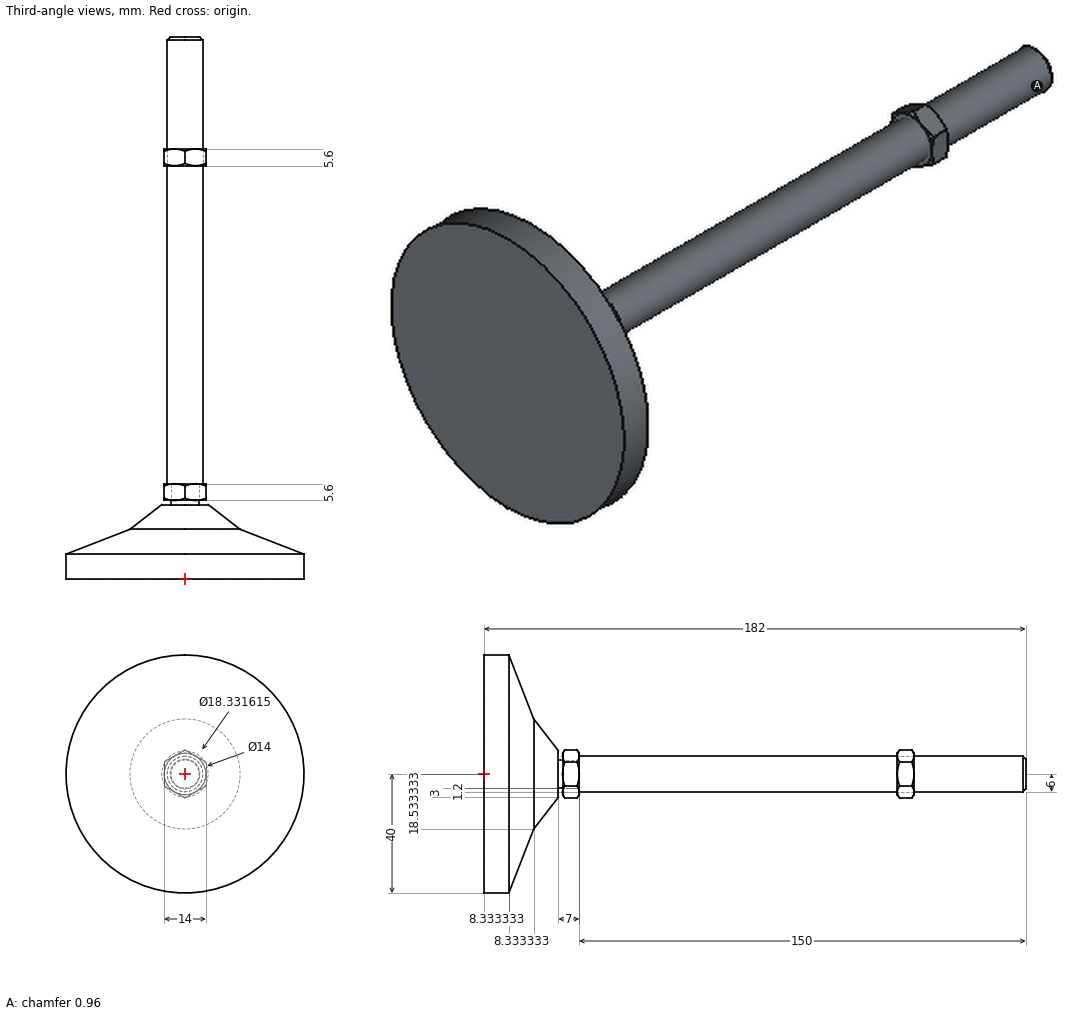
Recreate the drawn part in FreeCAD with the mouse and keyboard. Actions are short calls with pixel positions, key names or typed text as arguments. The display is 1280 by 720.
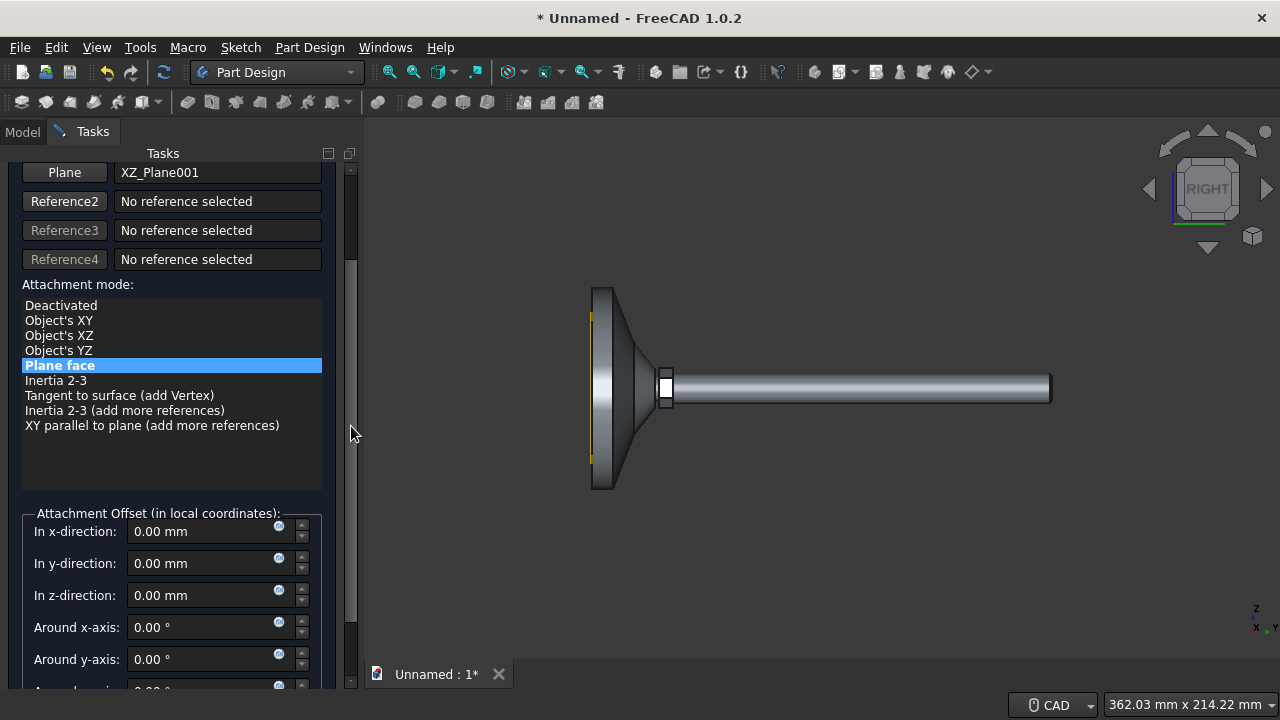
triple_click(210, 595)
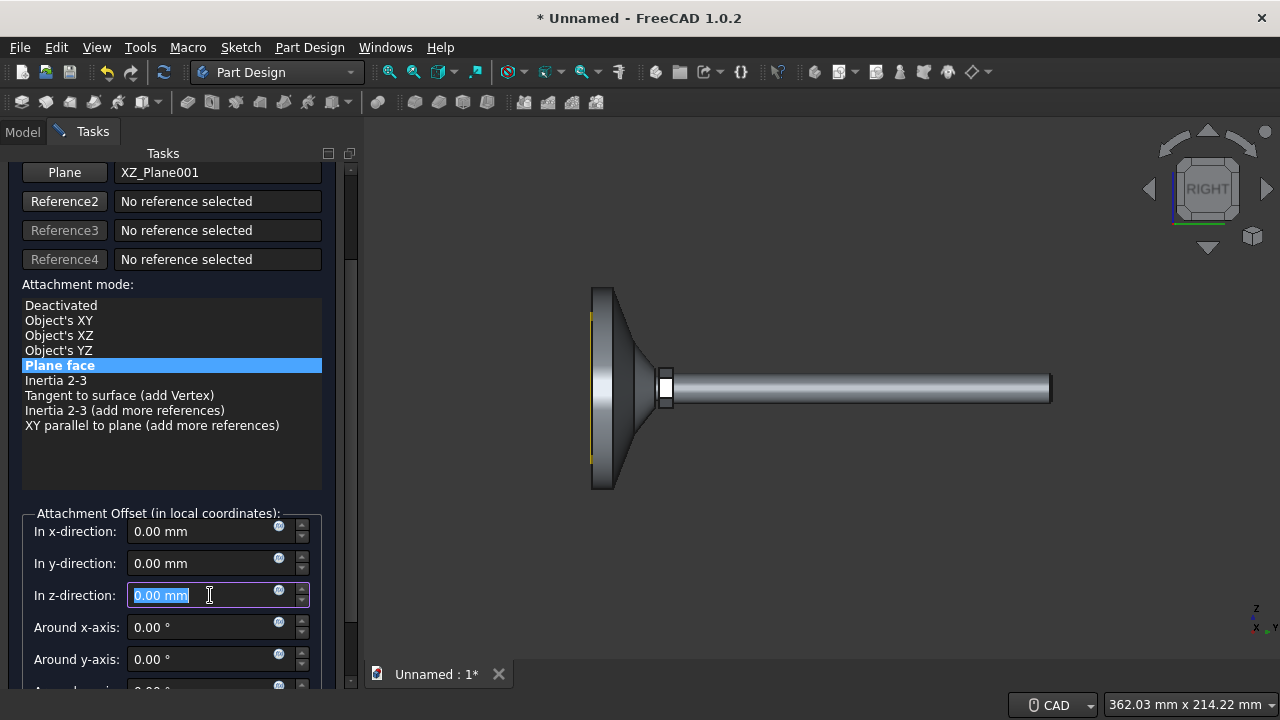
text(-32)
key(Tab)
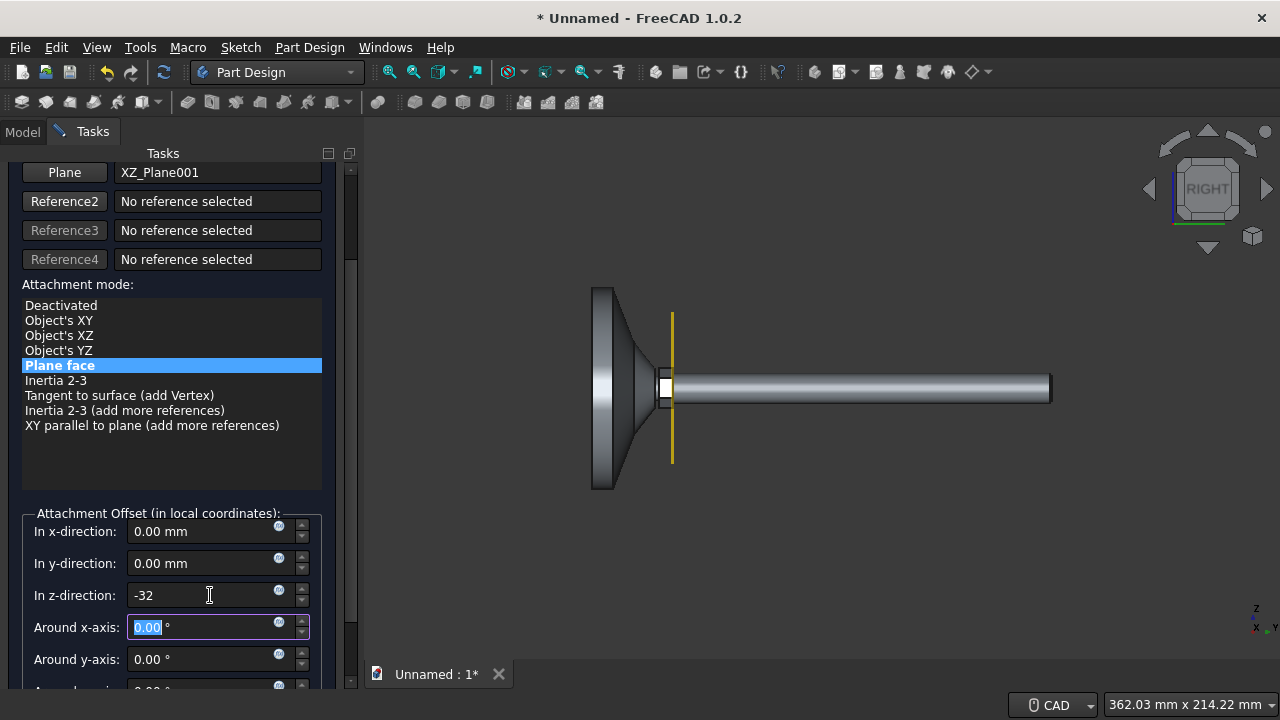
scroll(351, 426, up, 3)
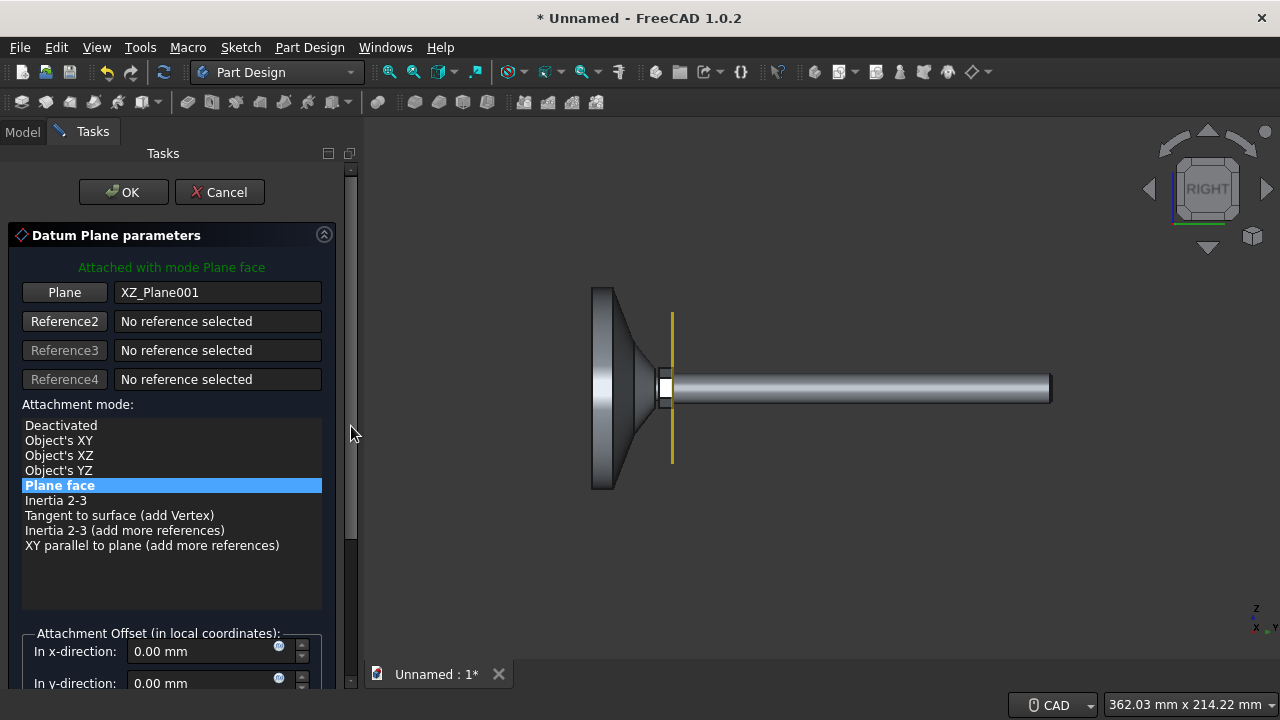
click(124, 192)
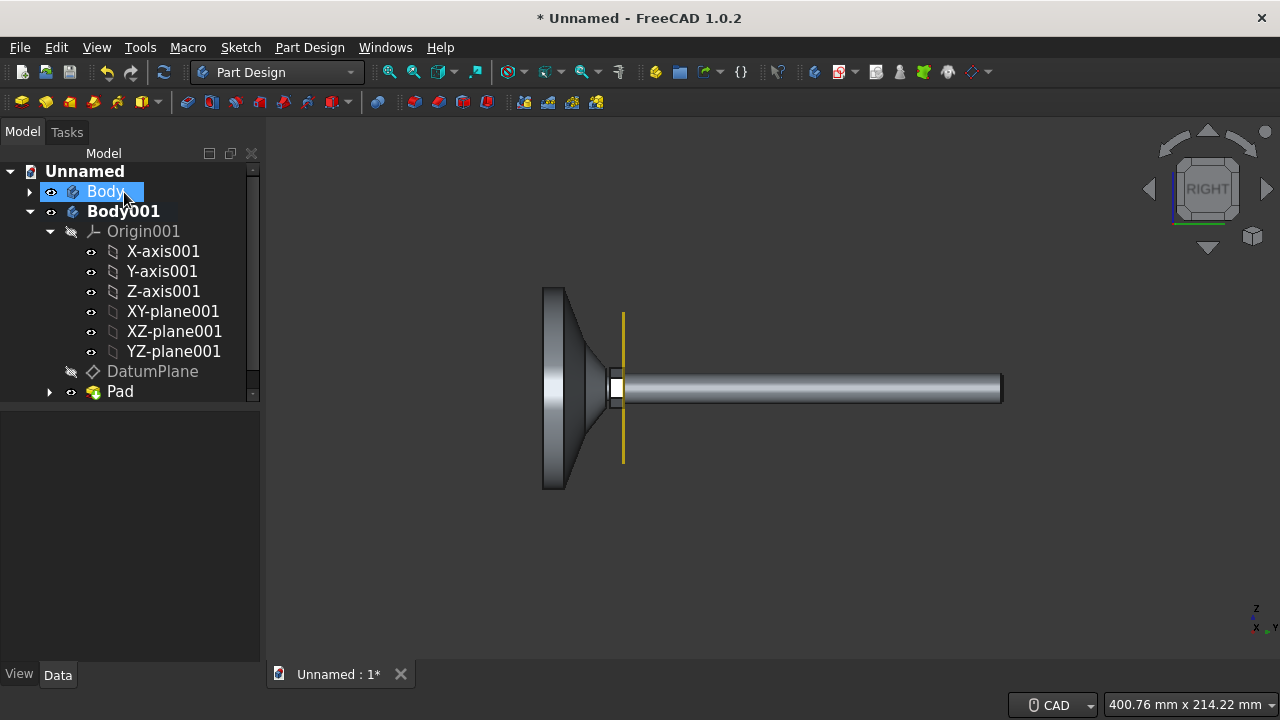
scroll(100, 287, down, 3)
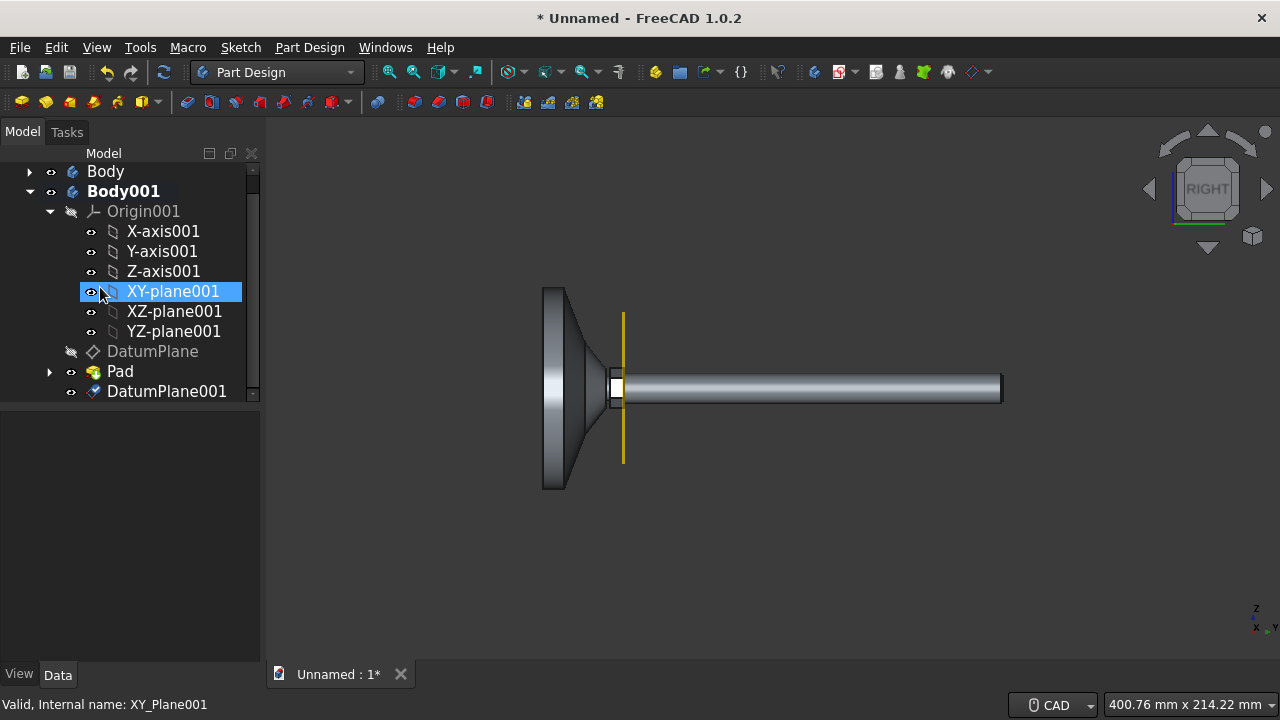
click(116, 392)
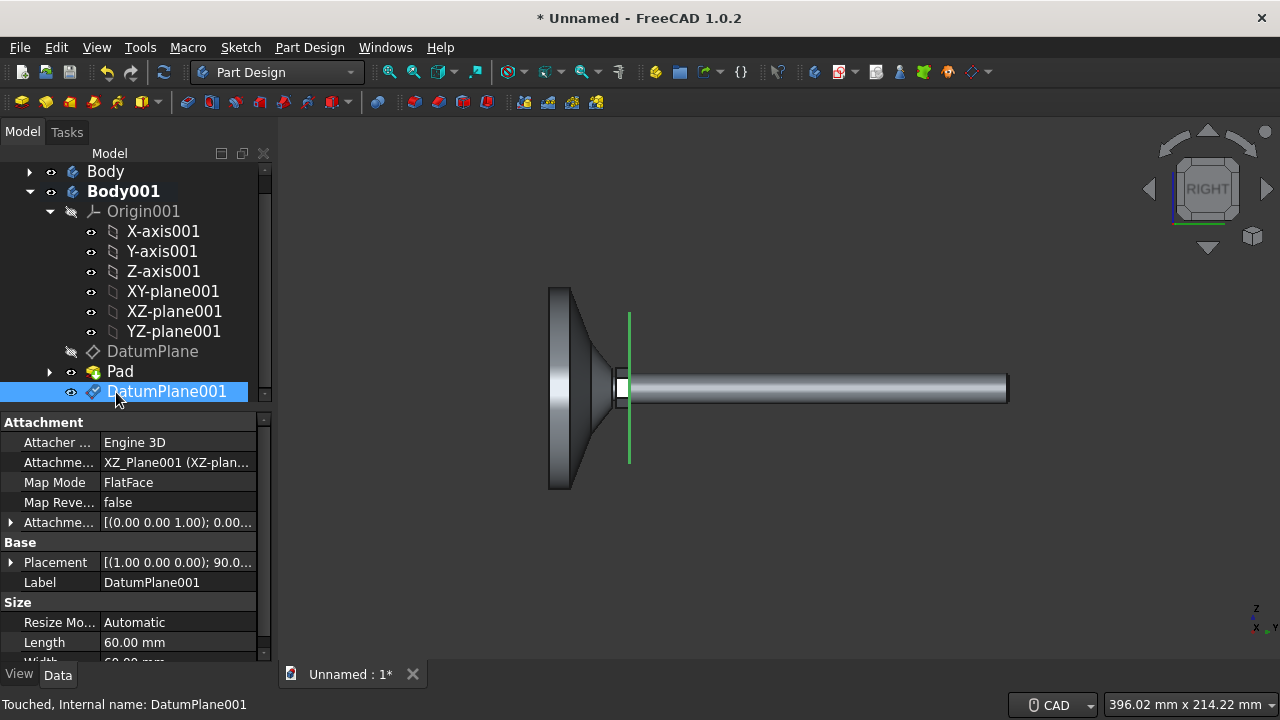
click(840, 72)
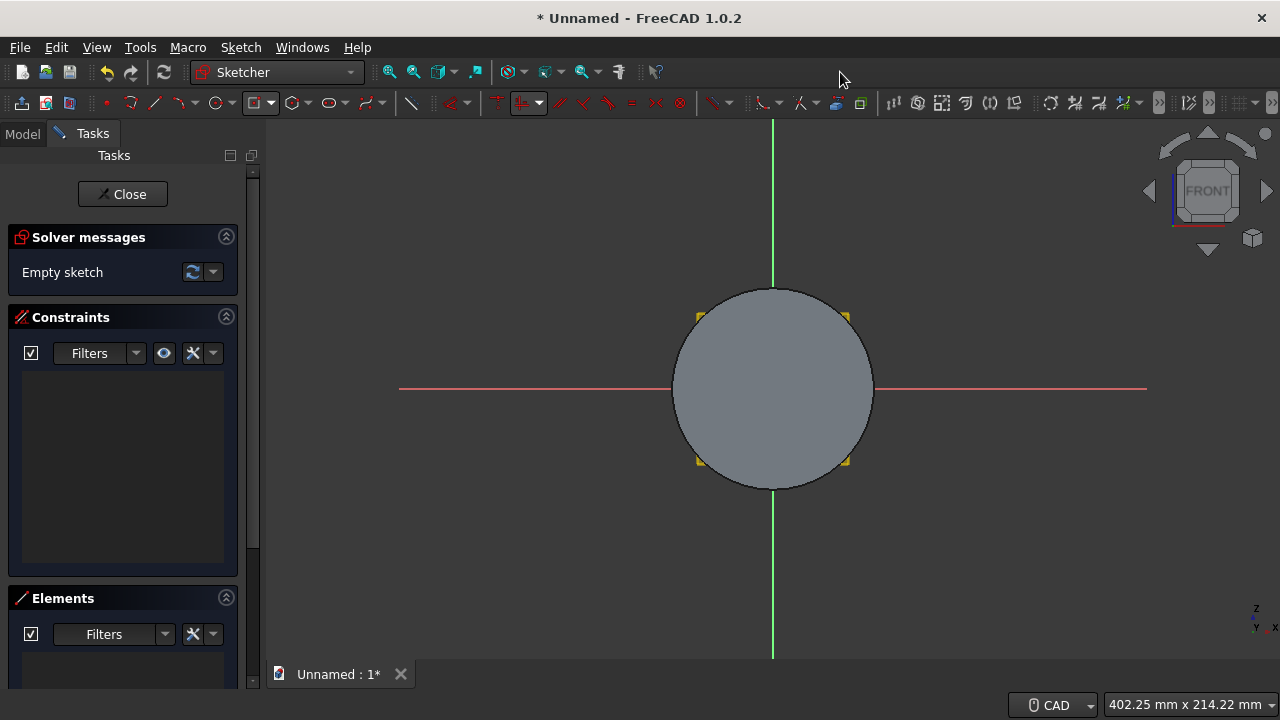
click(70, 104)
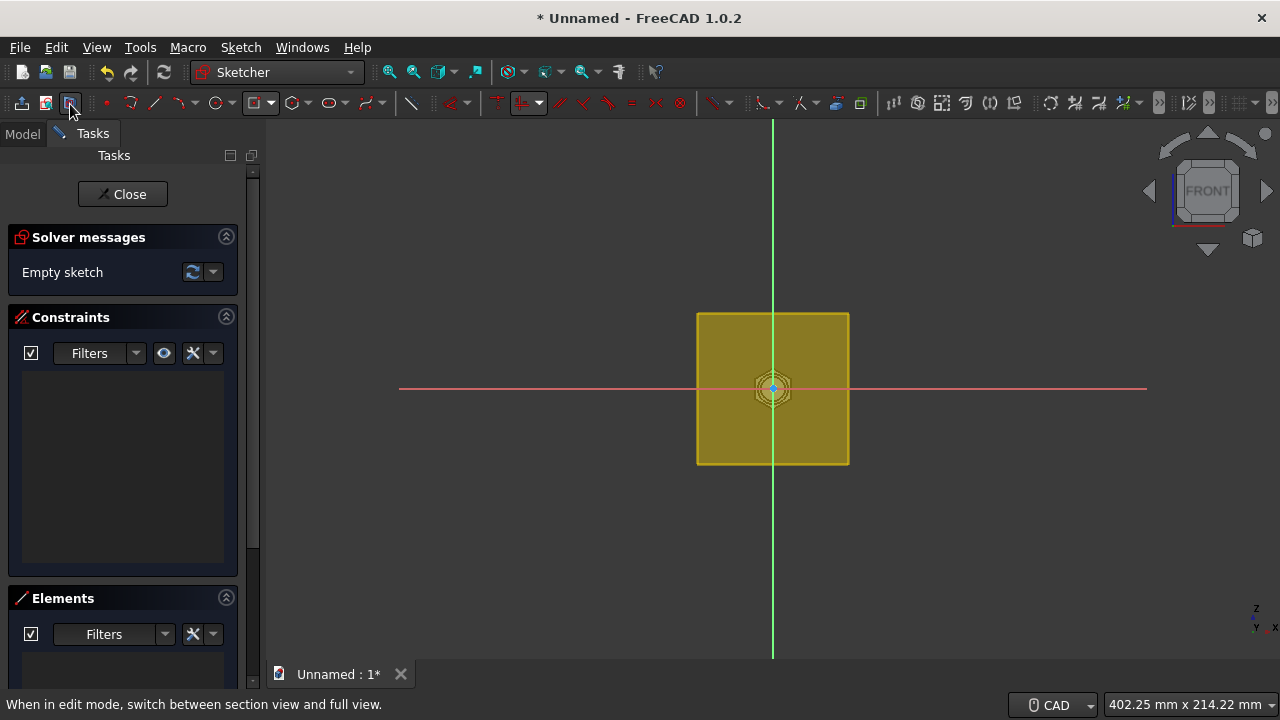
scroll(784, 389, up, 10)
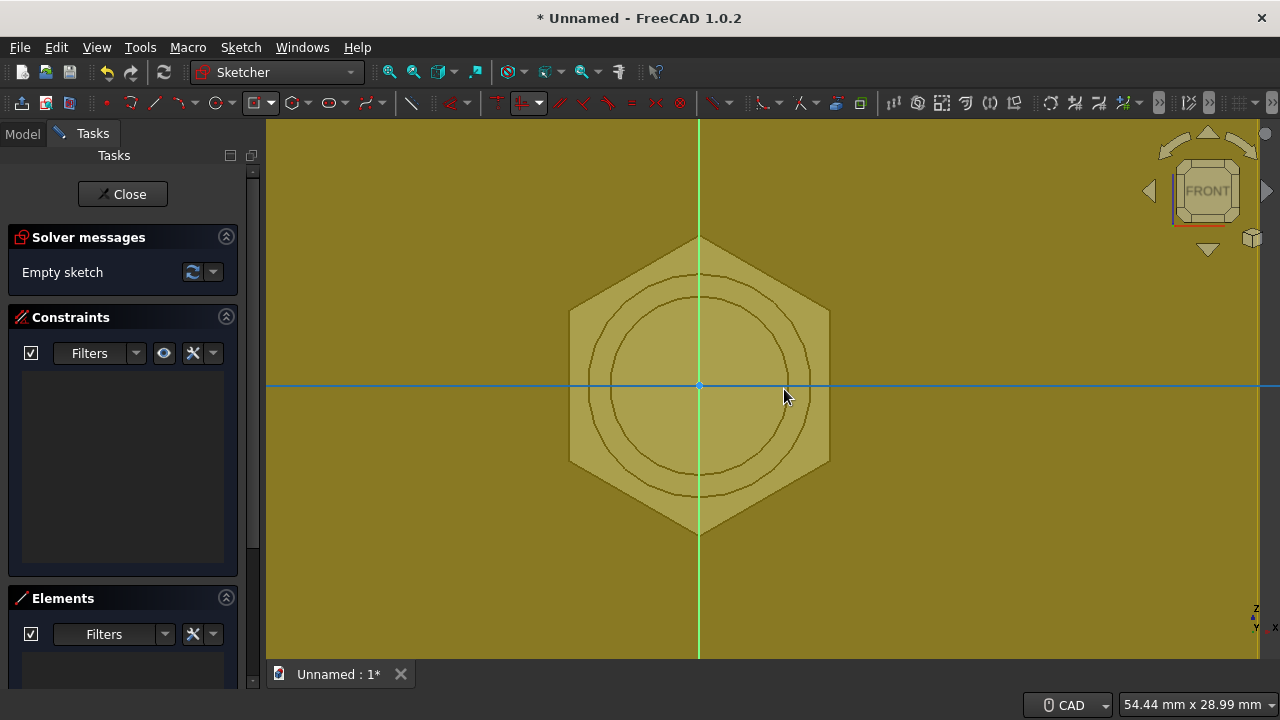
click(216, 104)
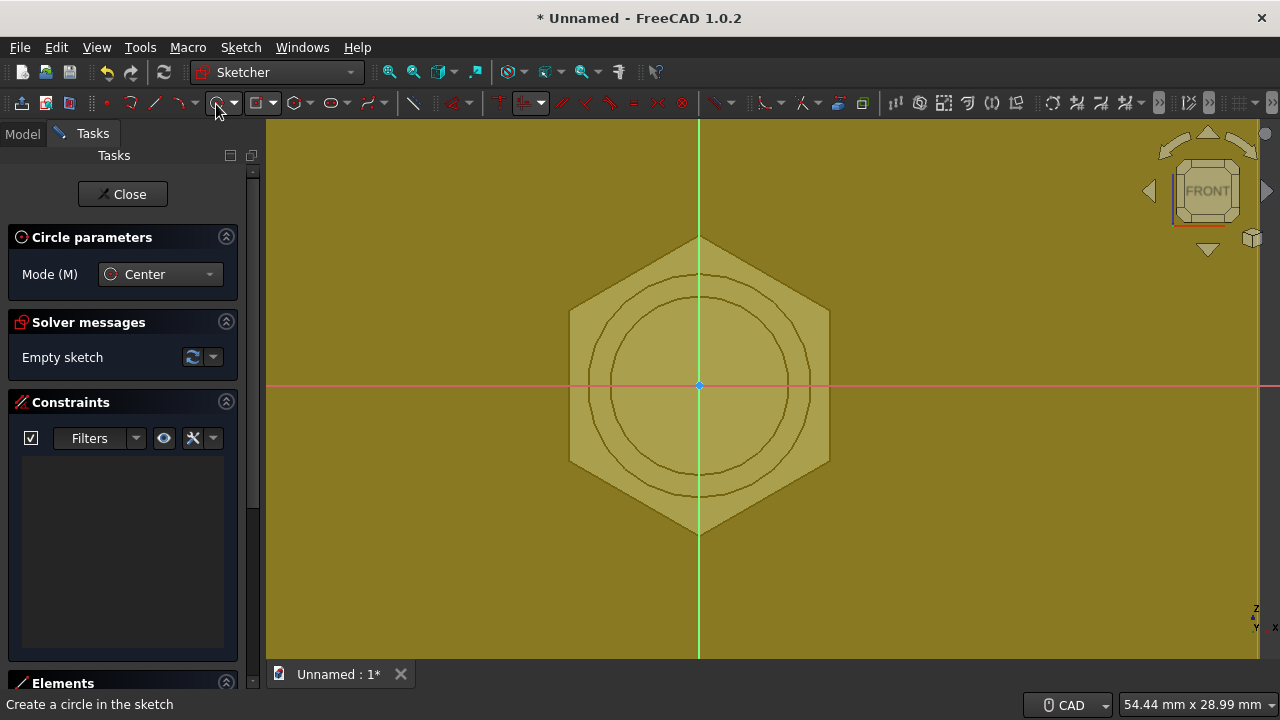
click(699, 386)
click(820, 265)